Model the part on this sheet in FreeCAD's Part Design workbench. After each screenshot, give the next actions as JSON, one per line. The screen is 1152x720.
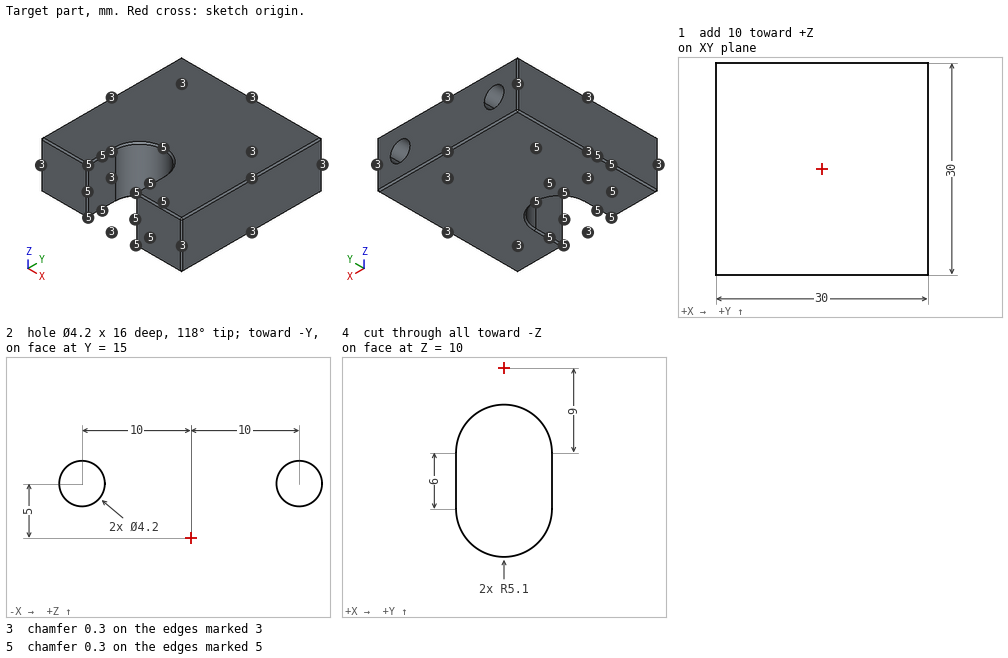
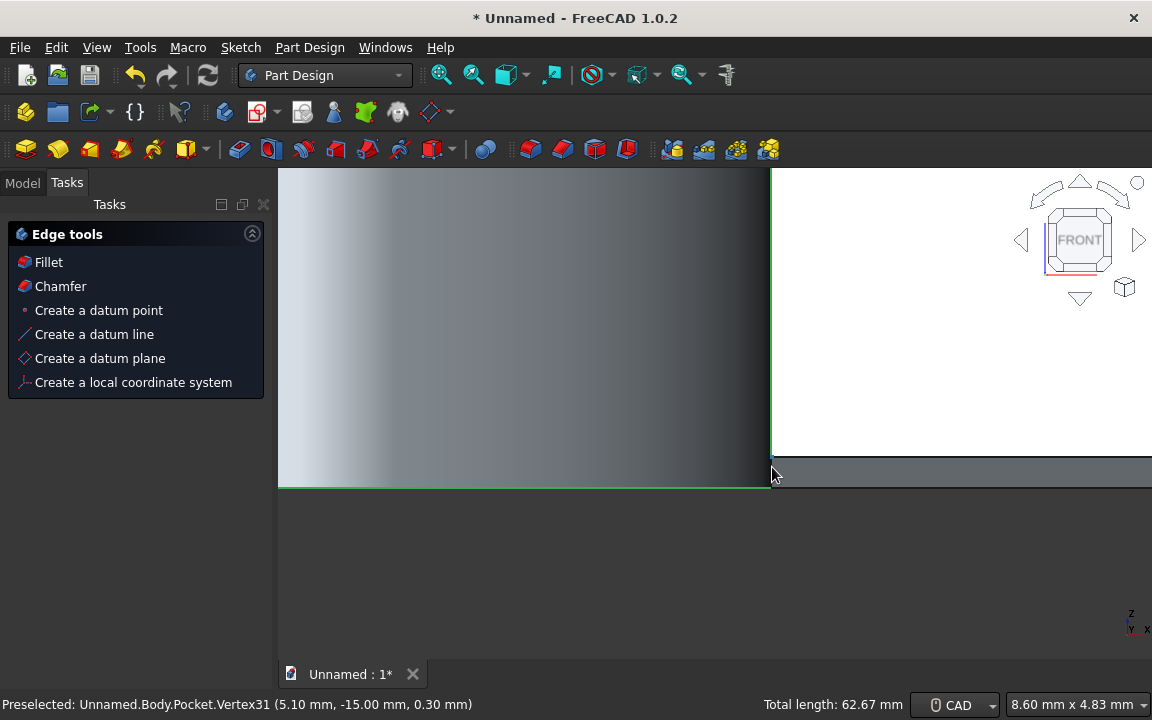
{"action": "left_click", "coordinate": [772, 471], "text": "ctrl"}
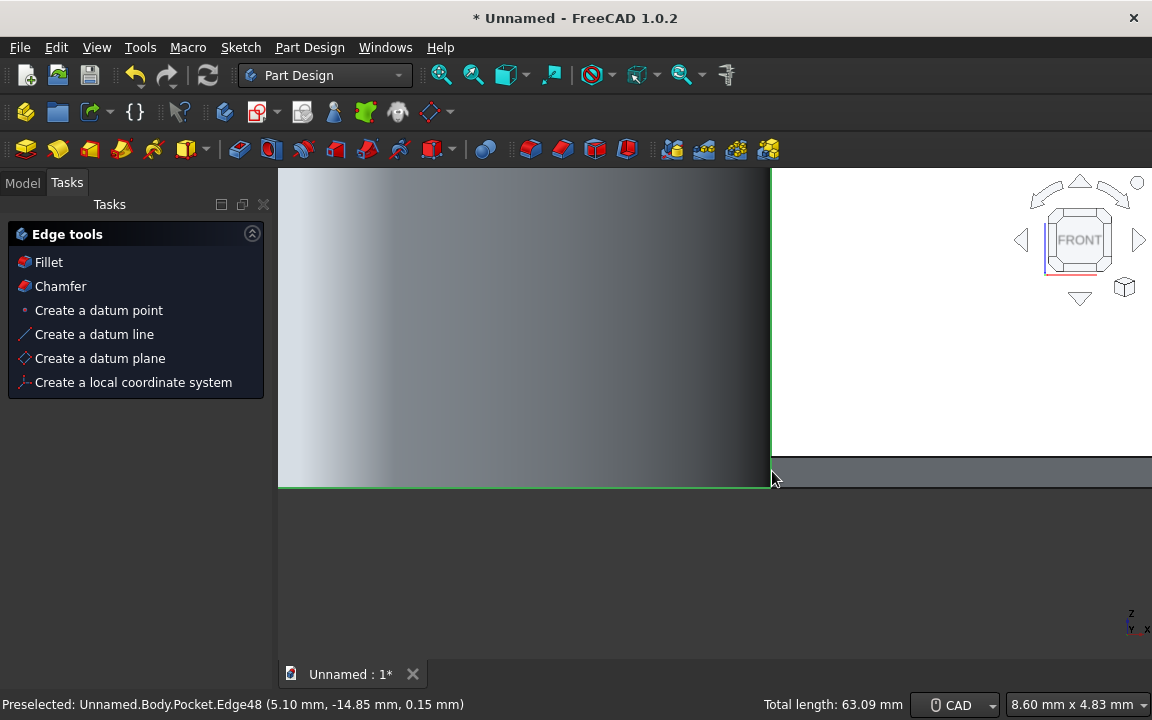
{"action": "left_click", "coordinate": [442, 76]}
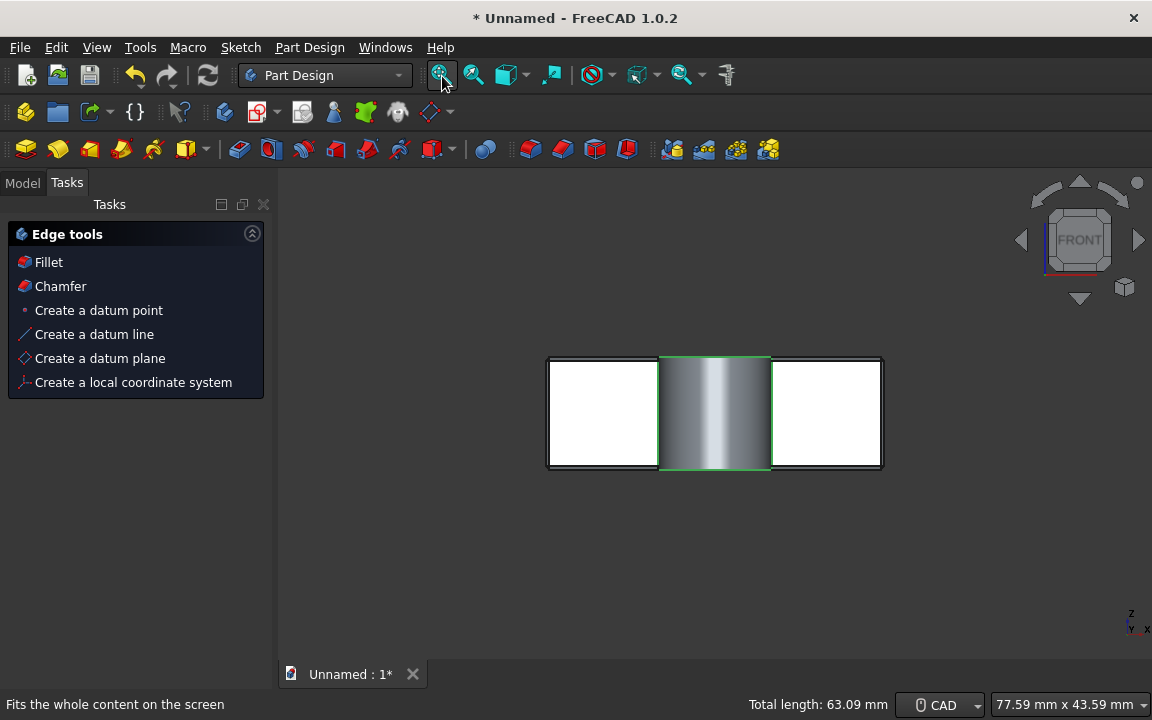
{"action": "key", "text": "3"}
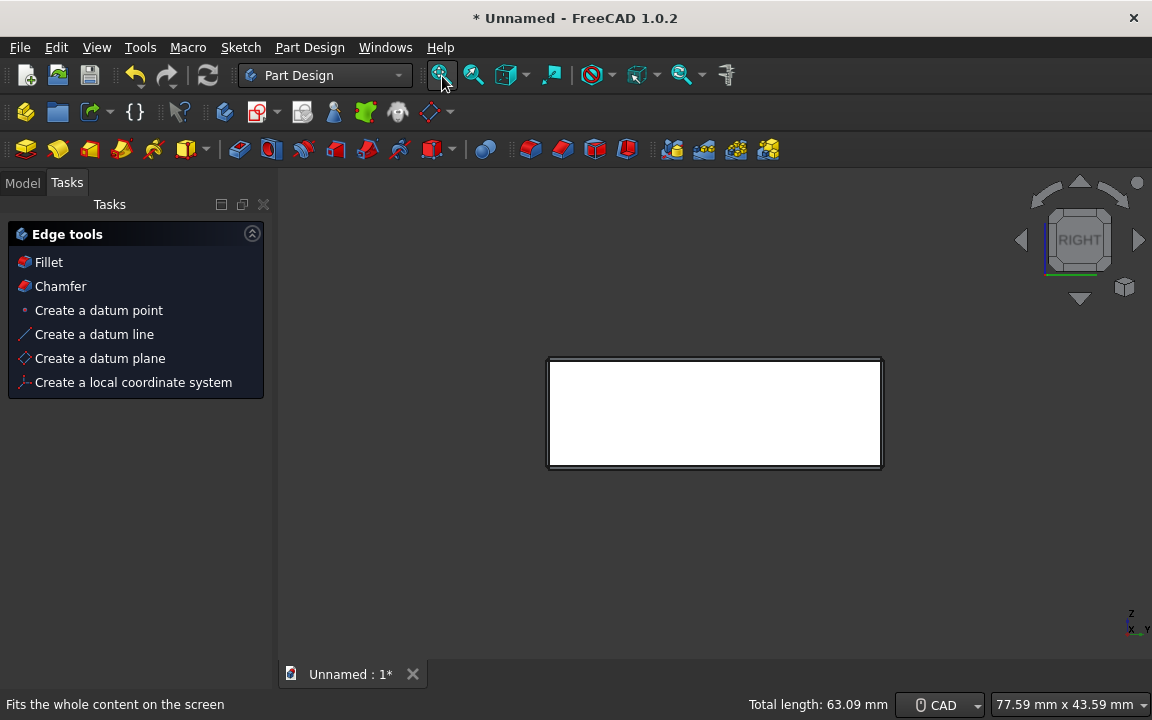
{"action": "left_click", "coordinate": [442, 76]}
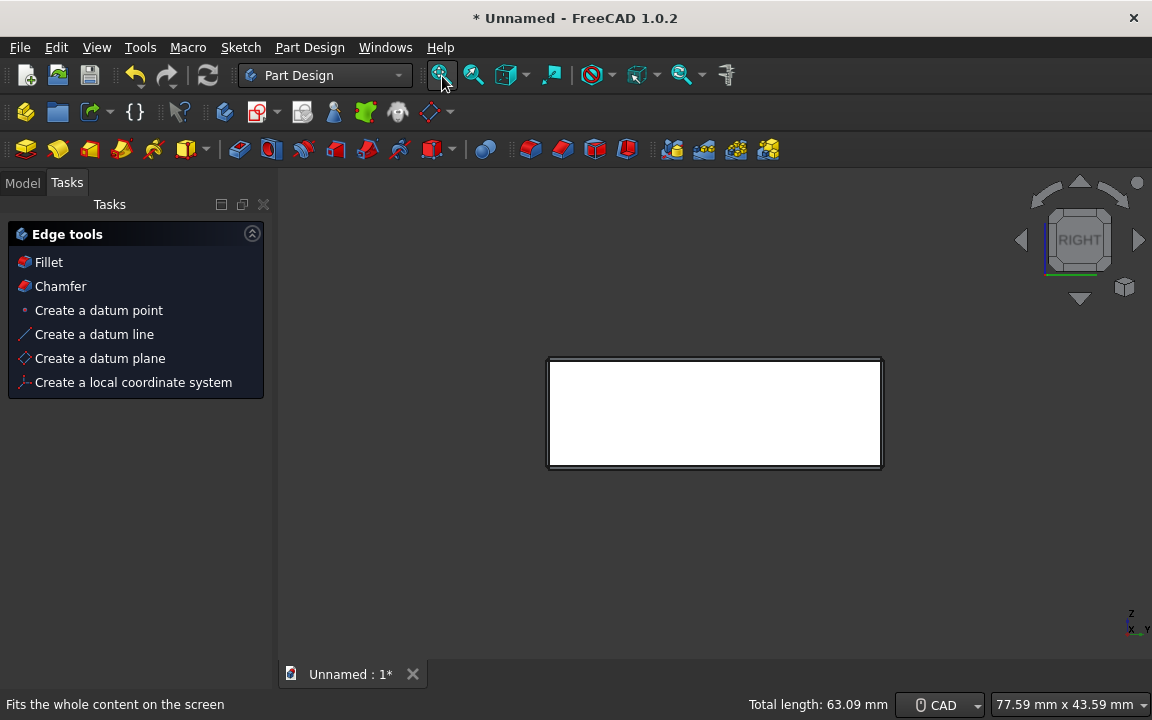
{"action": "scroll", "coordinate": [548, 467], "scroll_direction": "up", "scroll_amount": 11}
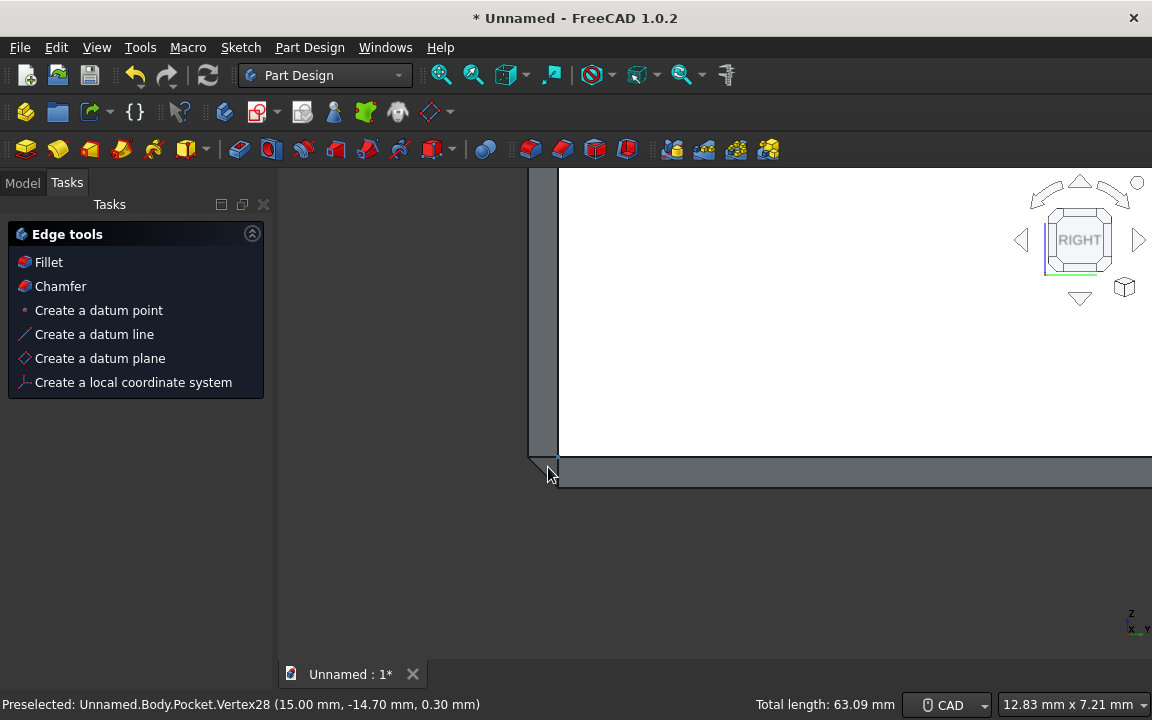
{"action": "left_click", "coordinate": [442, 76]}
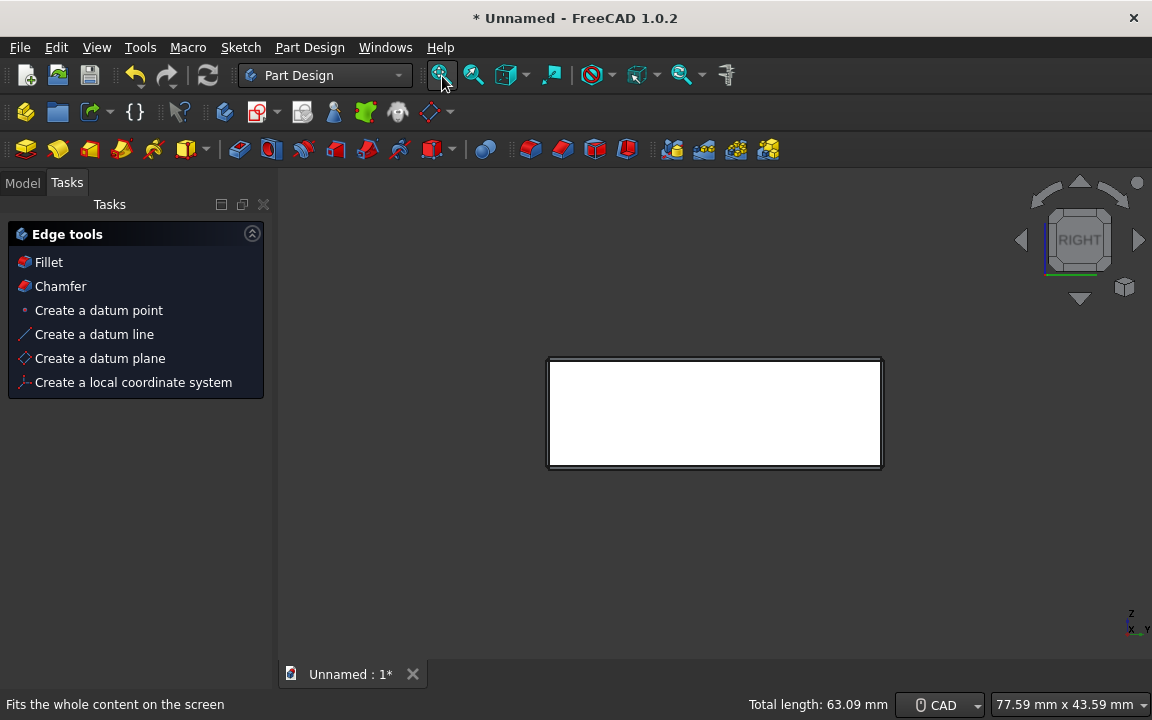
{"action": "key", "text": "5"}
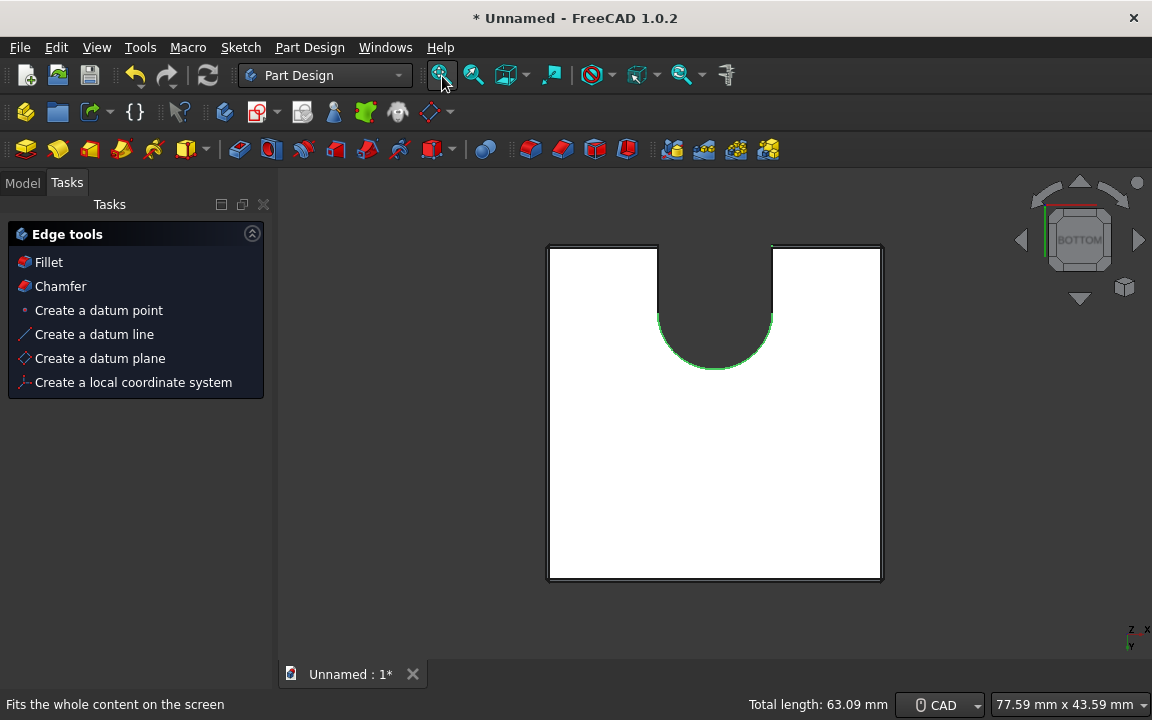
{"action": "left_click", "coordinate": [658, 279], "text": "ctrl"}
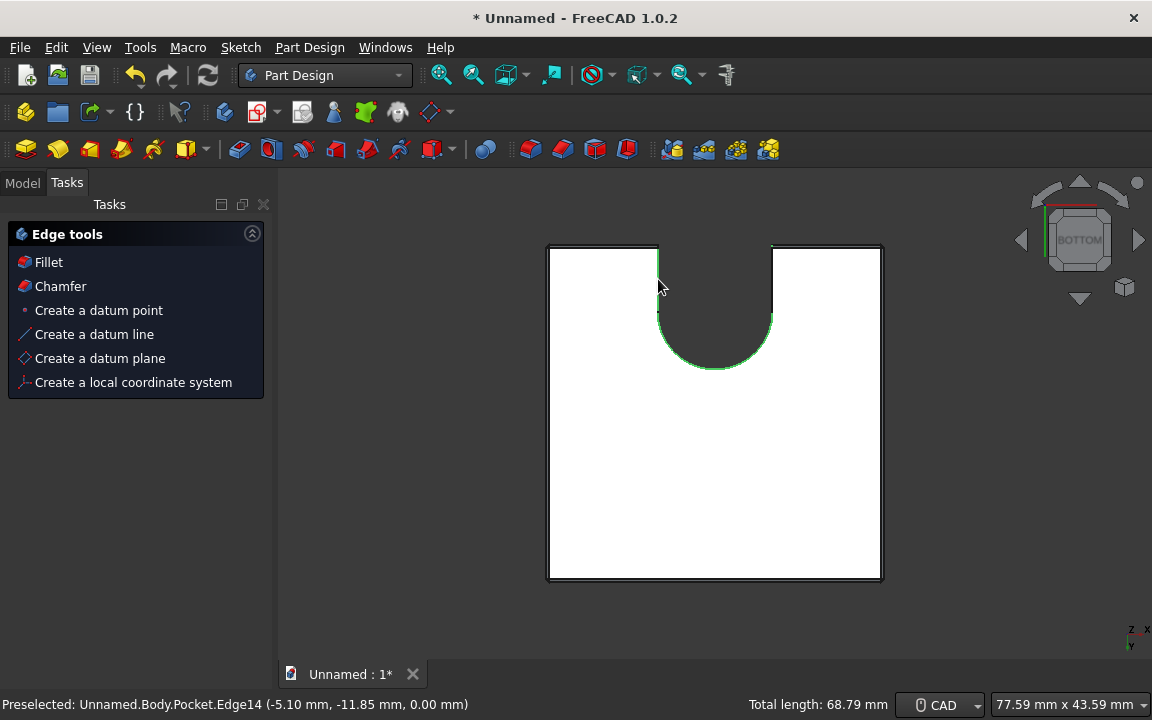
{"action": "left_click", "coordinate": [772, 279], "text": "ctrl"}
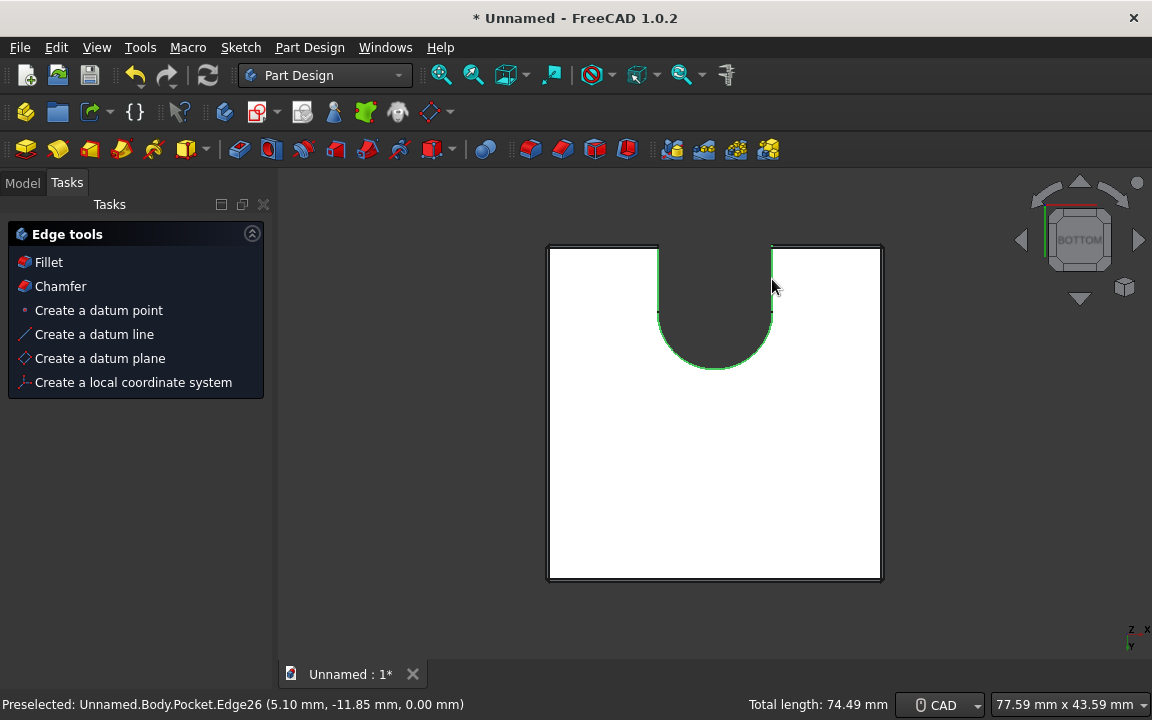
{"action": "scroll", "coordinate": [658, 245], "scroll_direction": "up", "scroll_amount": 11}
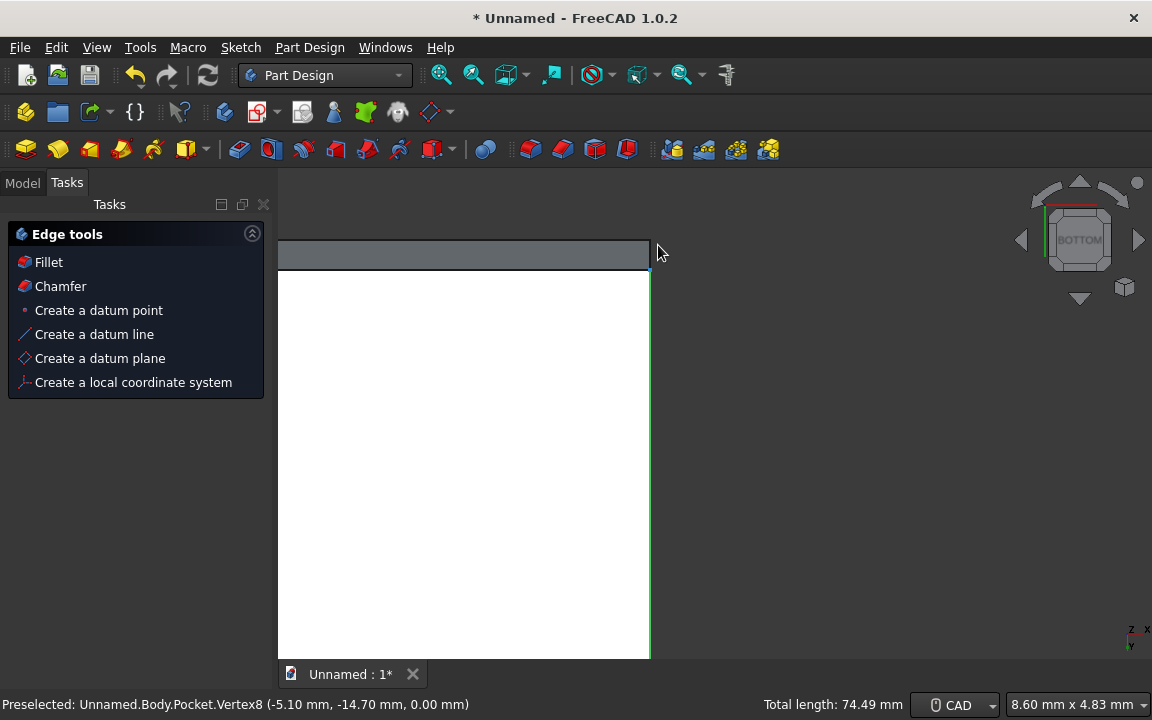
{"action": "left_click", "coordinate": [650, 254], "text": "ctrl"}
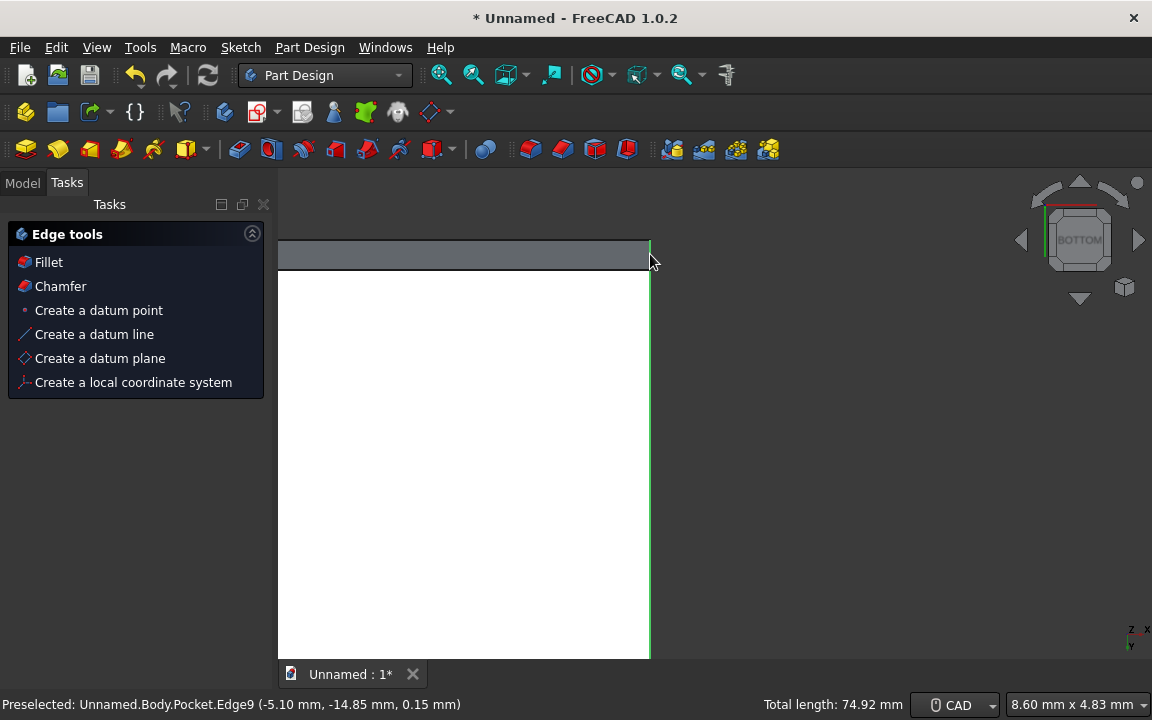
{"action": "left_click", "coordinate": [442, 76]}